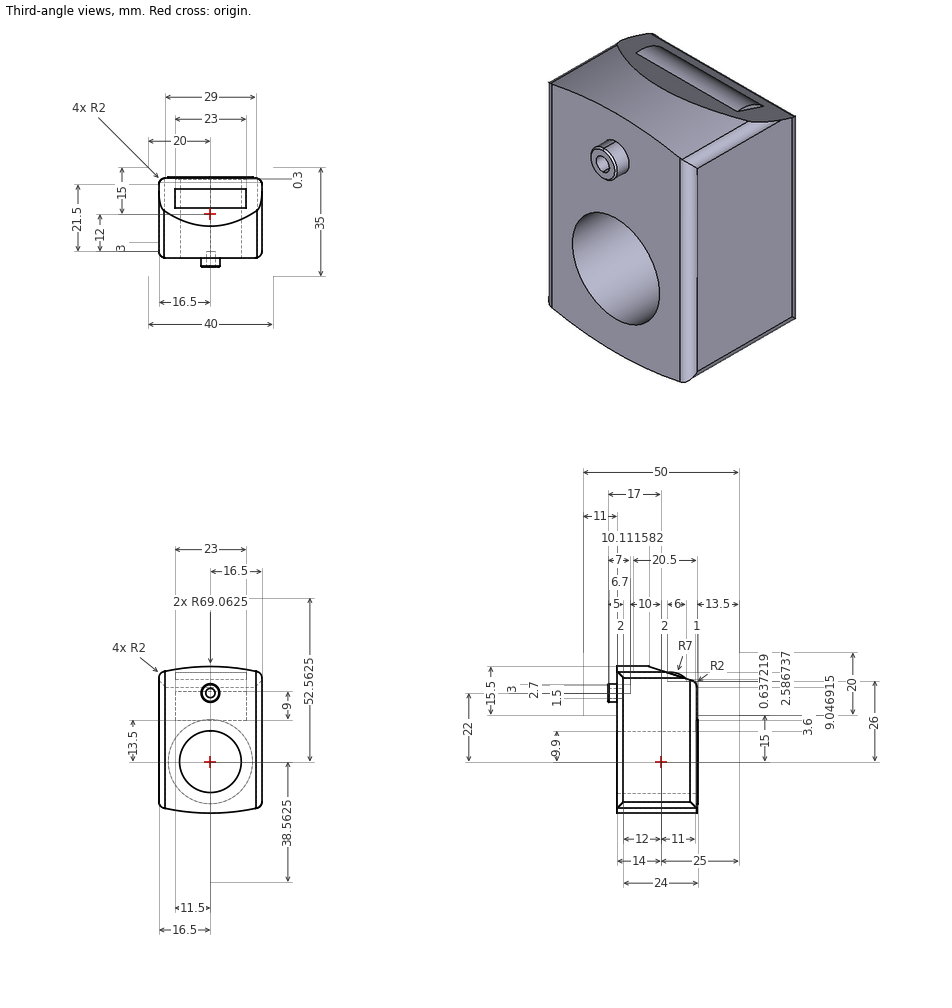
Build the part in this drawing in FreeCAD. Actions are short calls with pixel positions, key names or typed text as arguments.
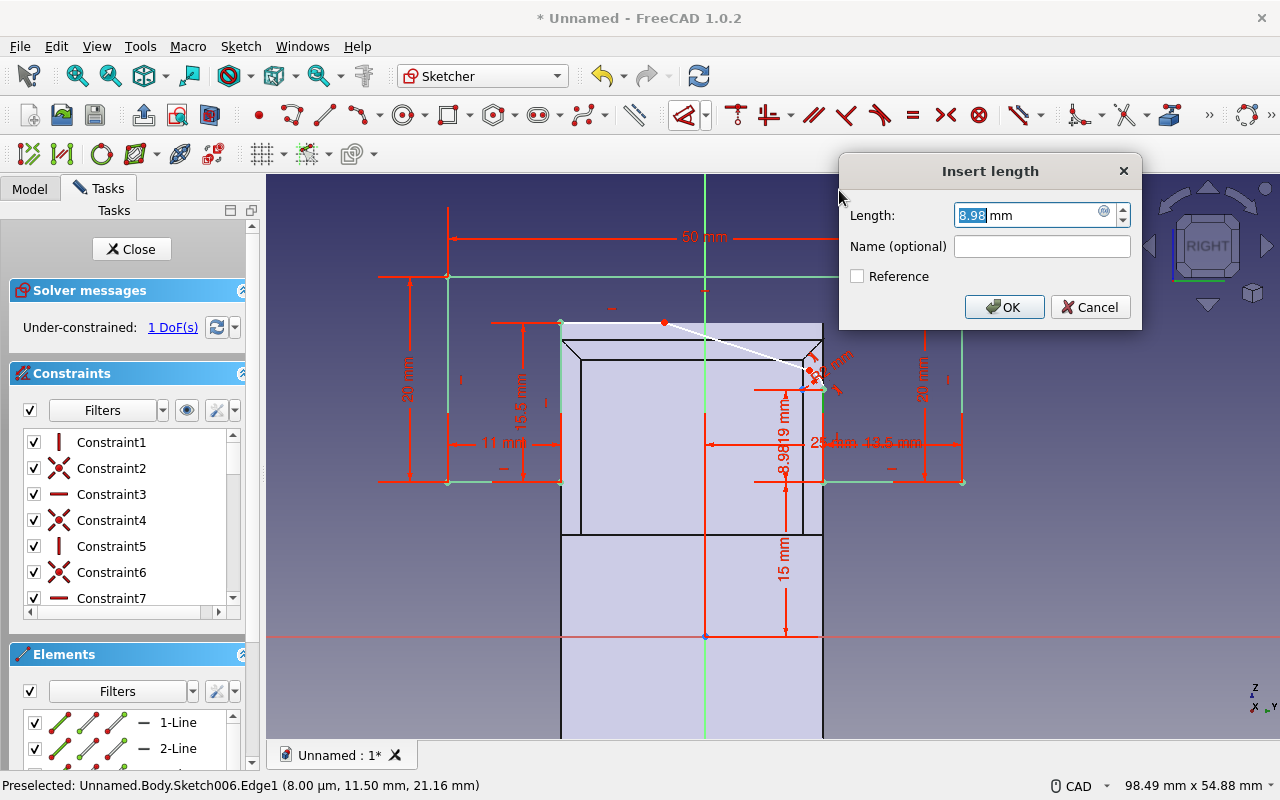
text(9.046915)
key(Return)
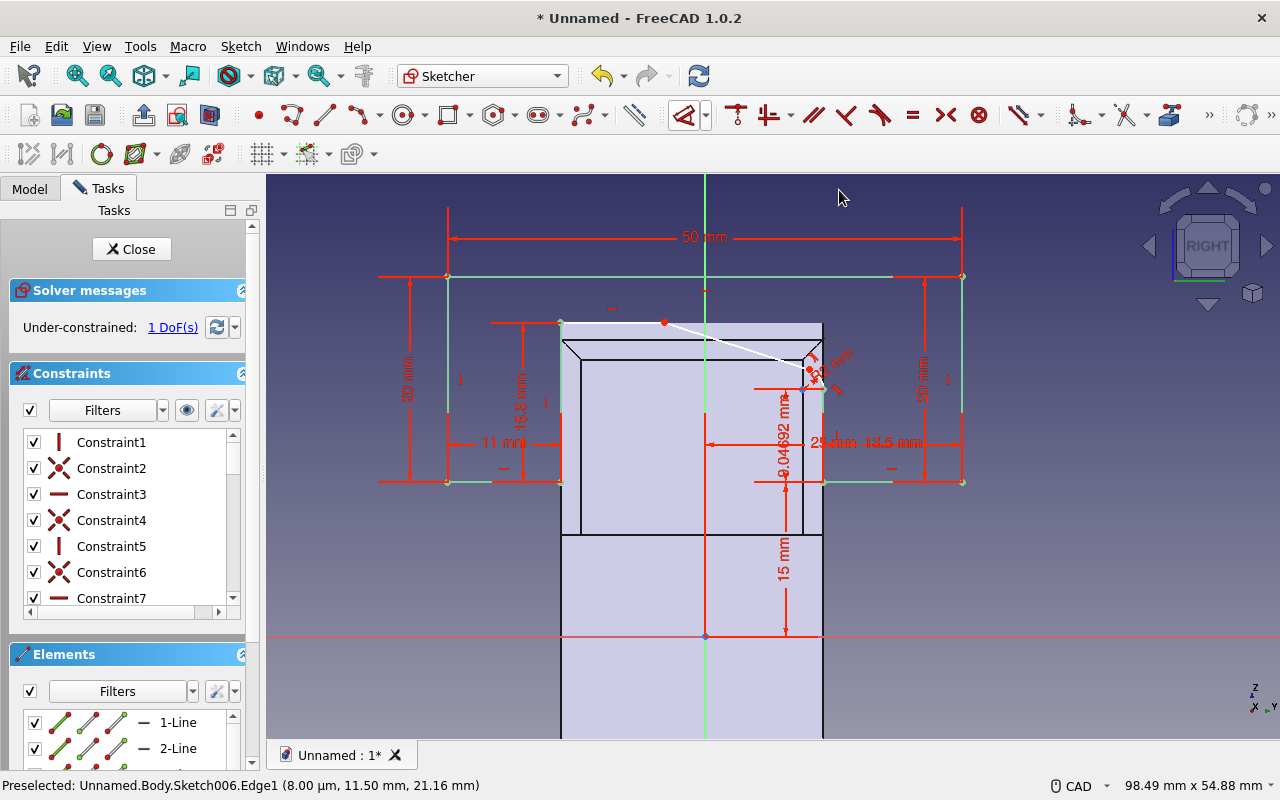
click(592, 323)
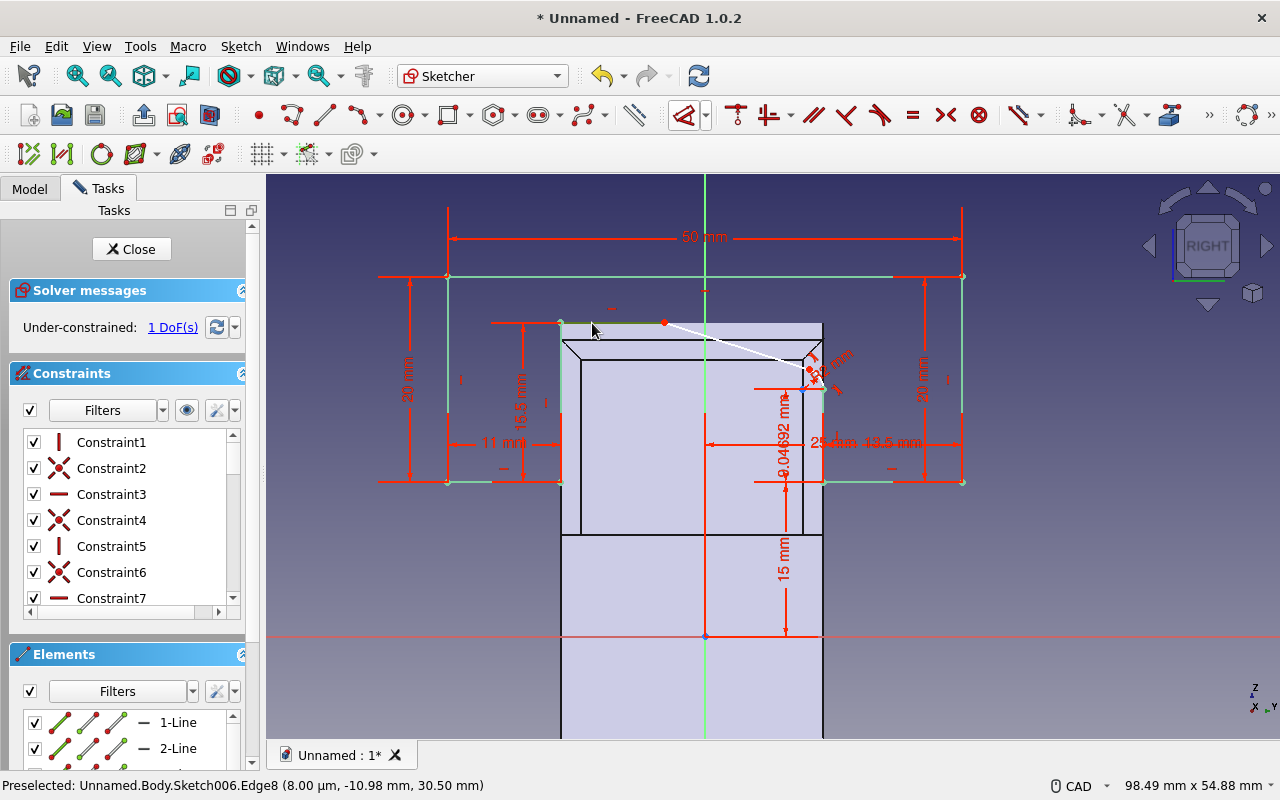
click(706, 116)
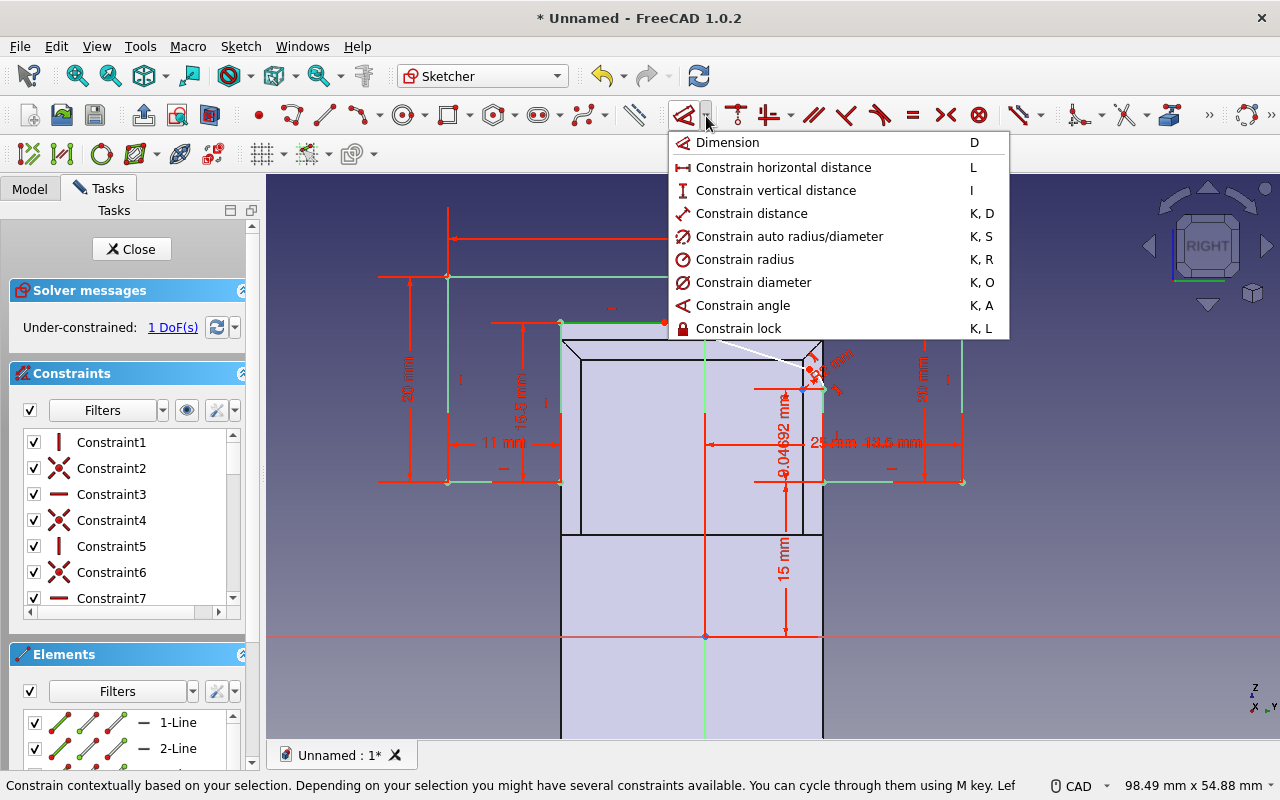
click(839, 168)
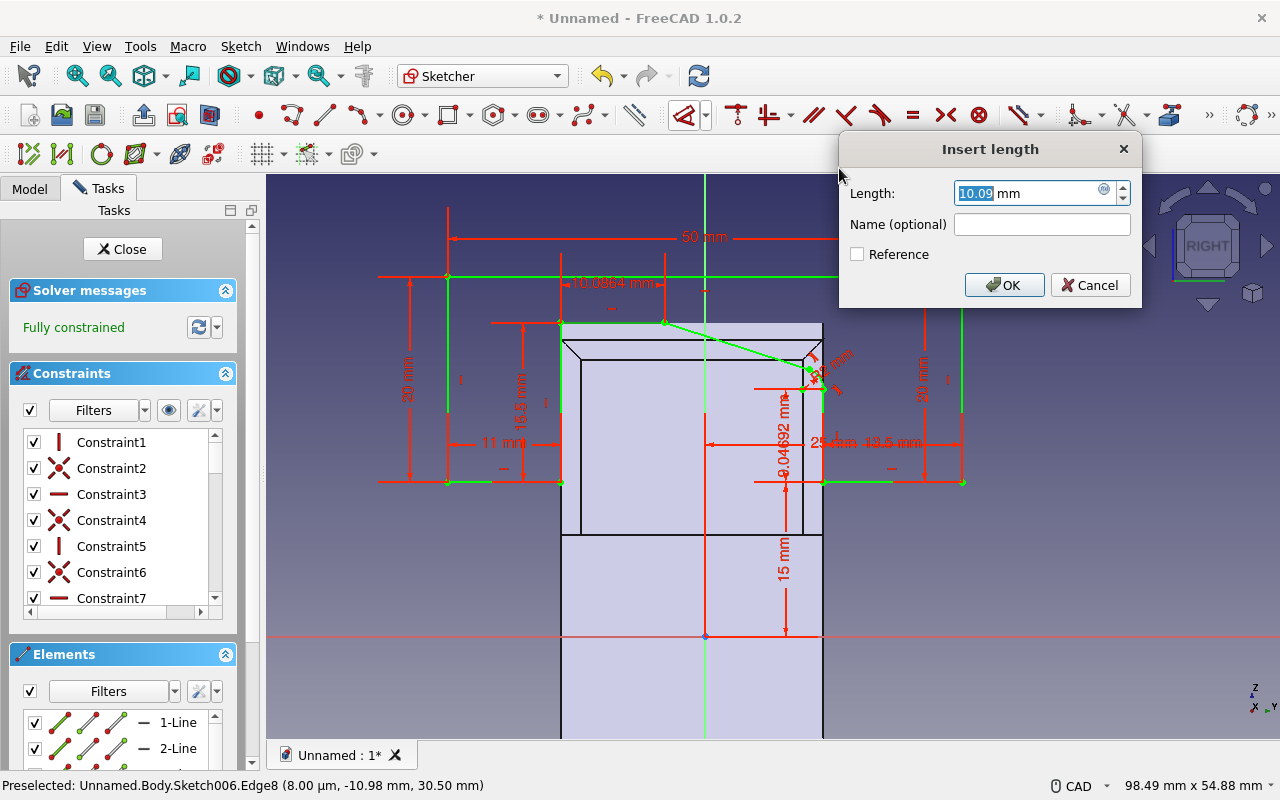
text(10.111582)
key(Return)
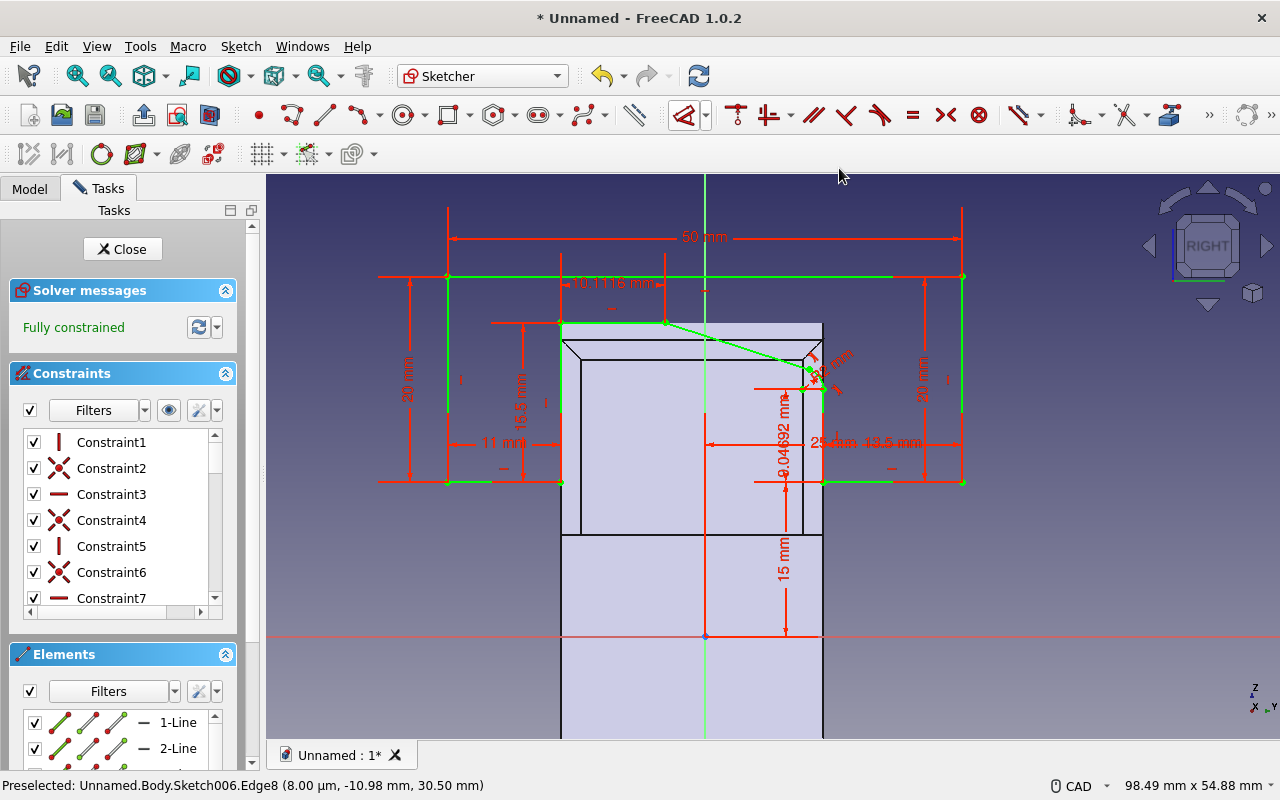
click(123, 249)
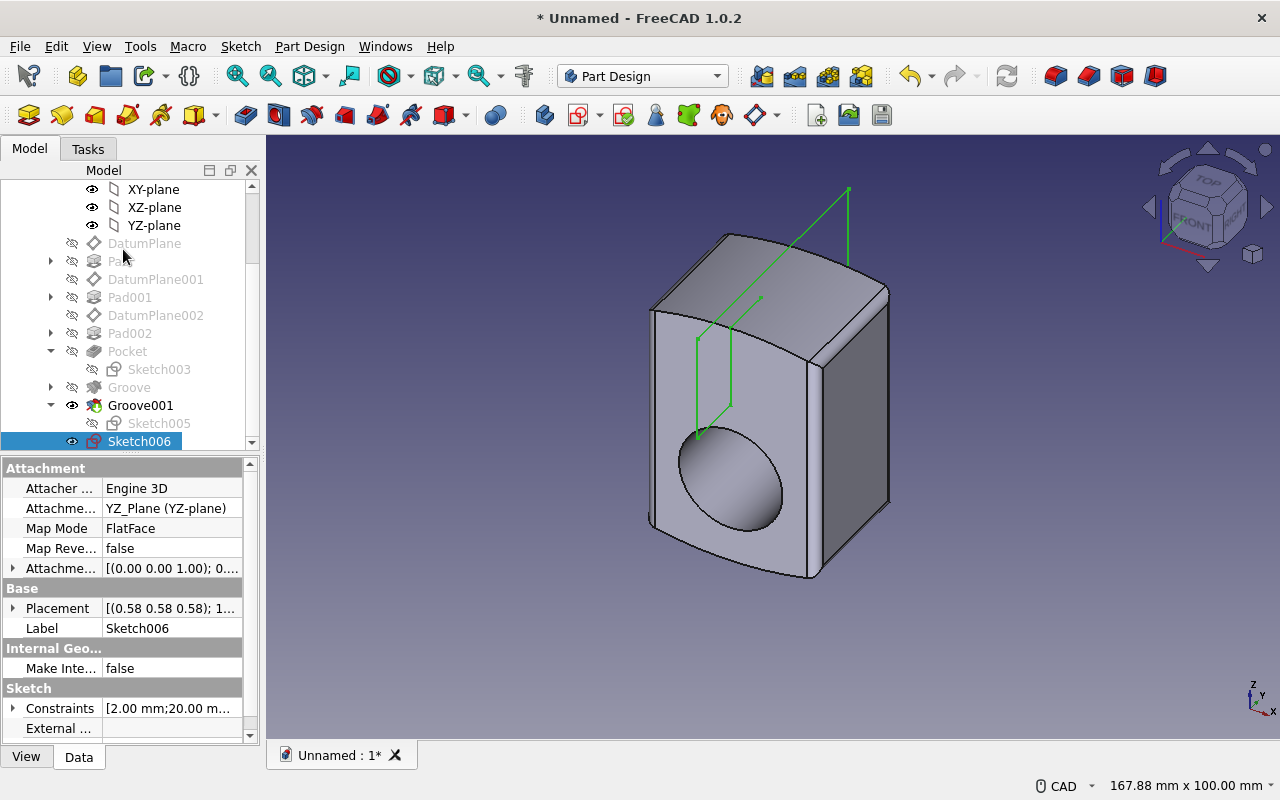
click(246, 116)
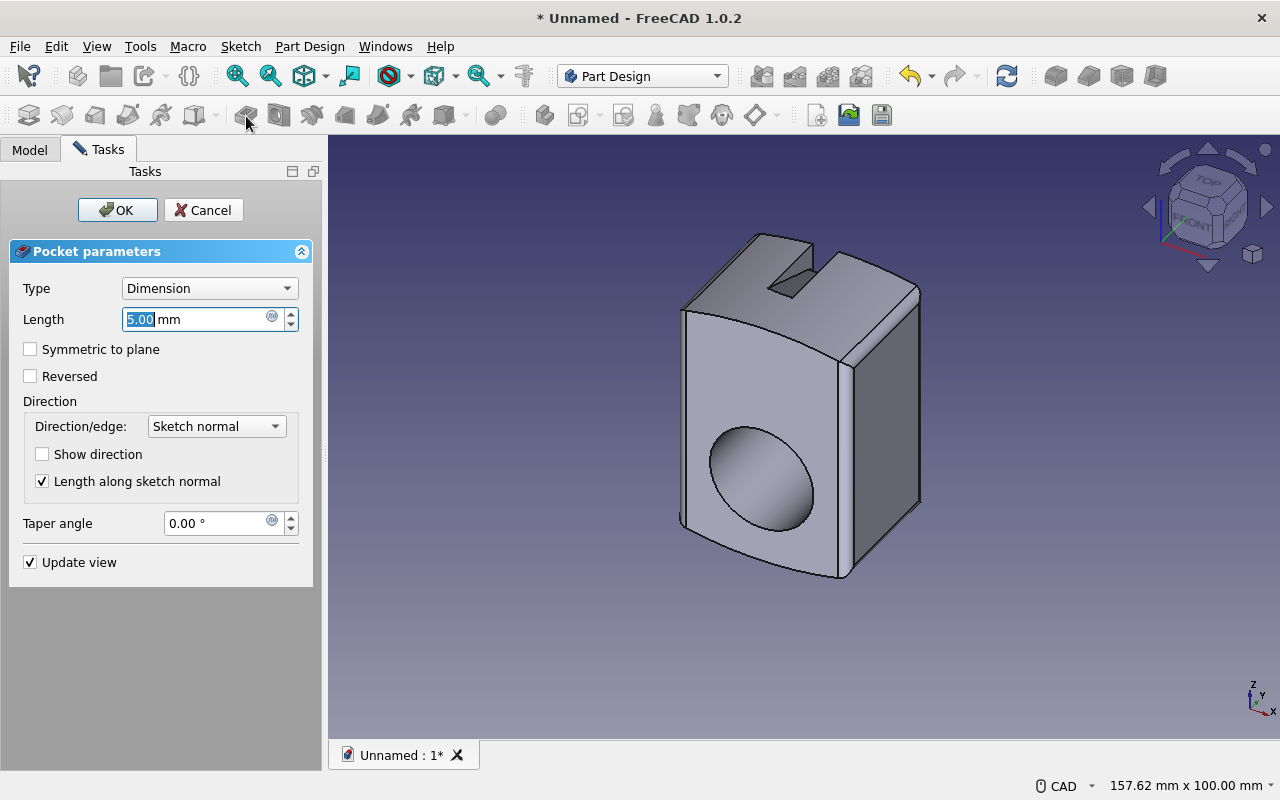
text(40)
key(Tab)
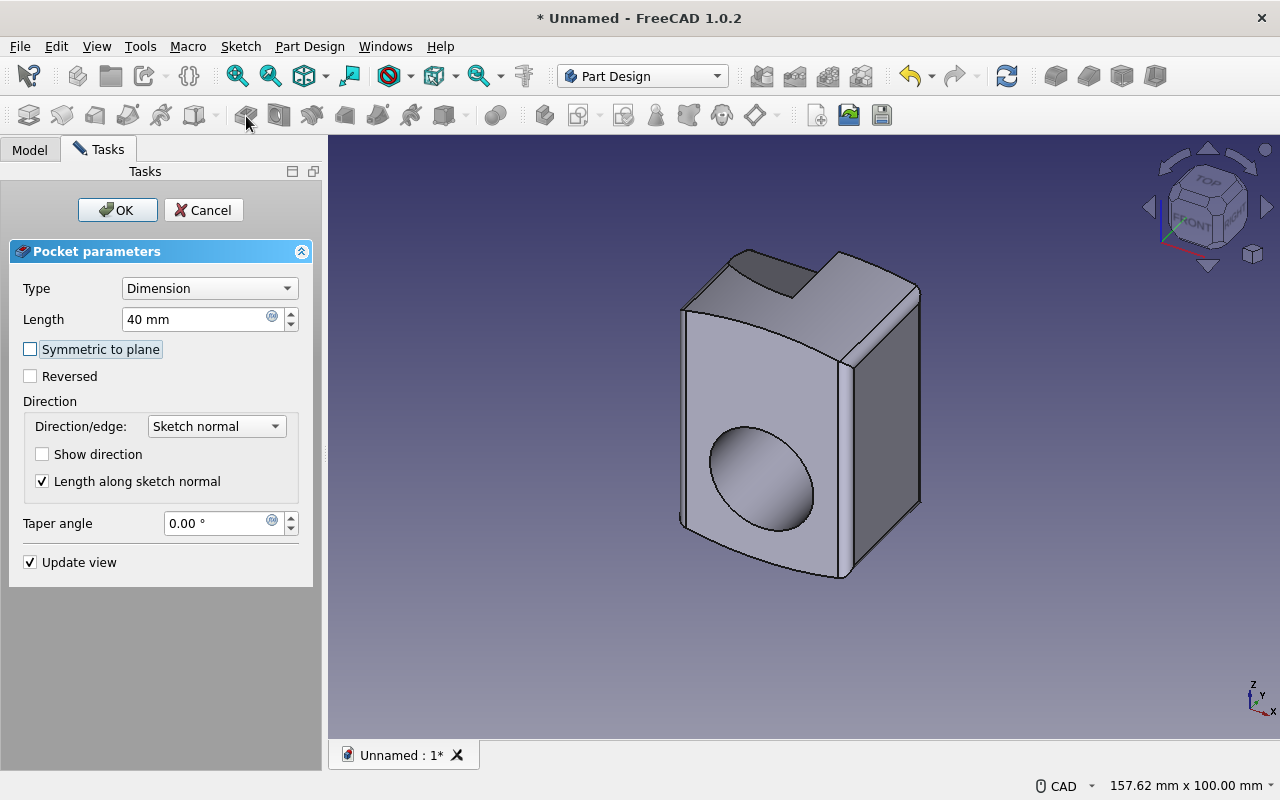
click(31, 349)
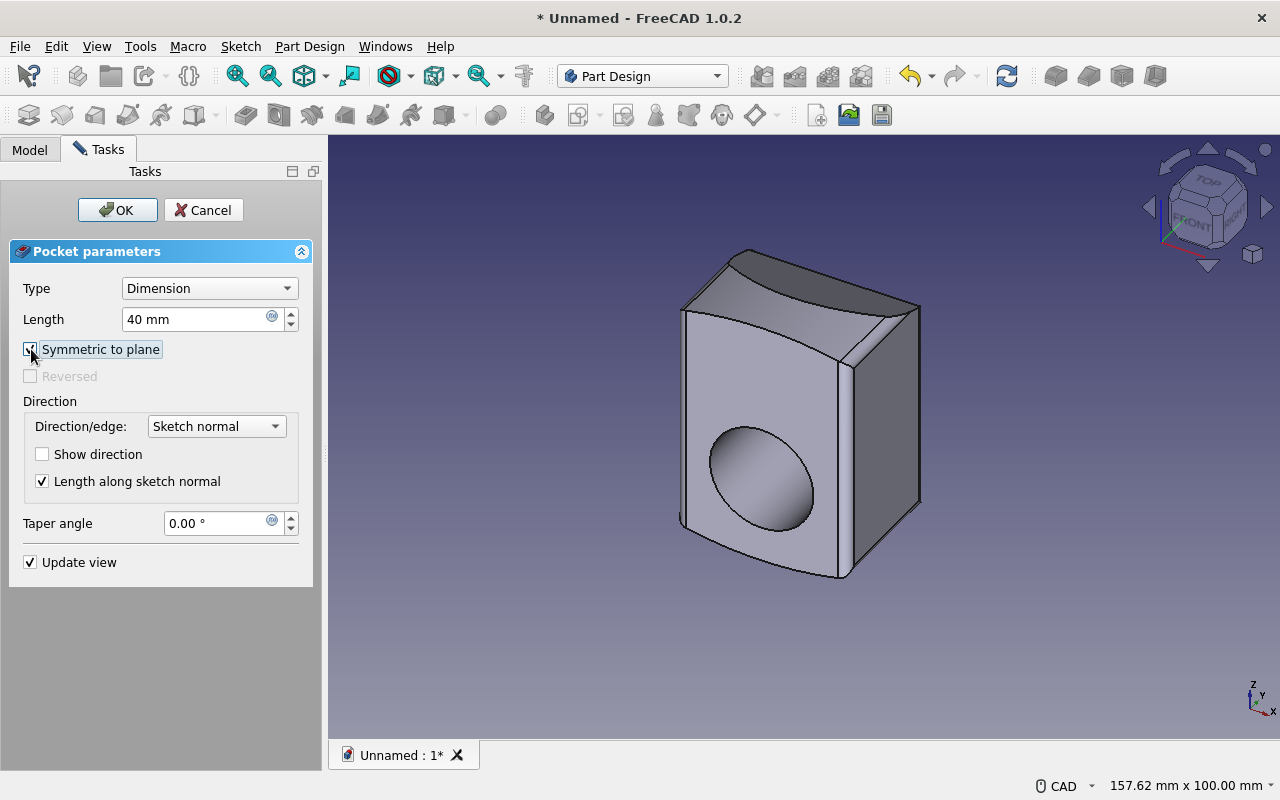
click(118, 210)